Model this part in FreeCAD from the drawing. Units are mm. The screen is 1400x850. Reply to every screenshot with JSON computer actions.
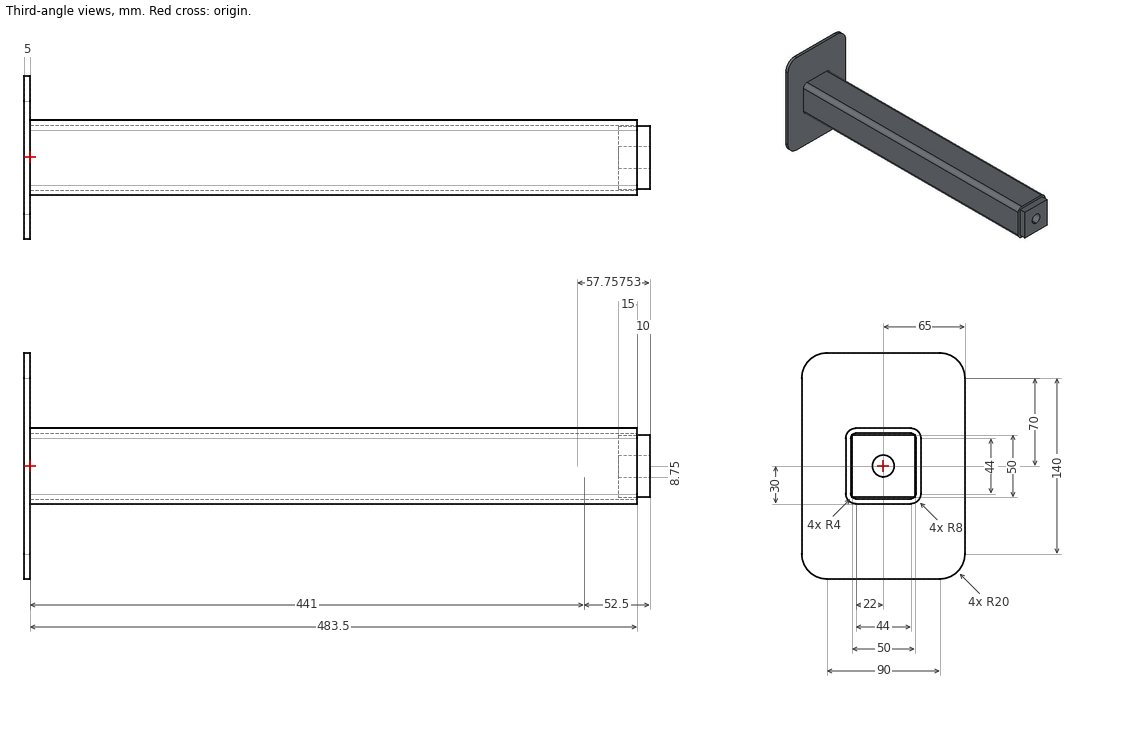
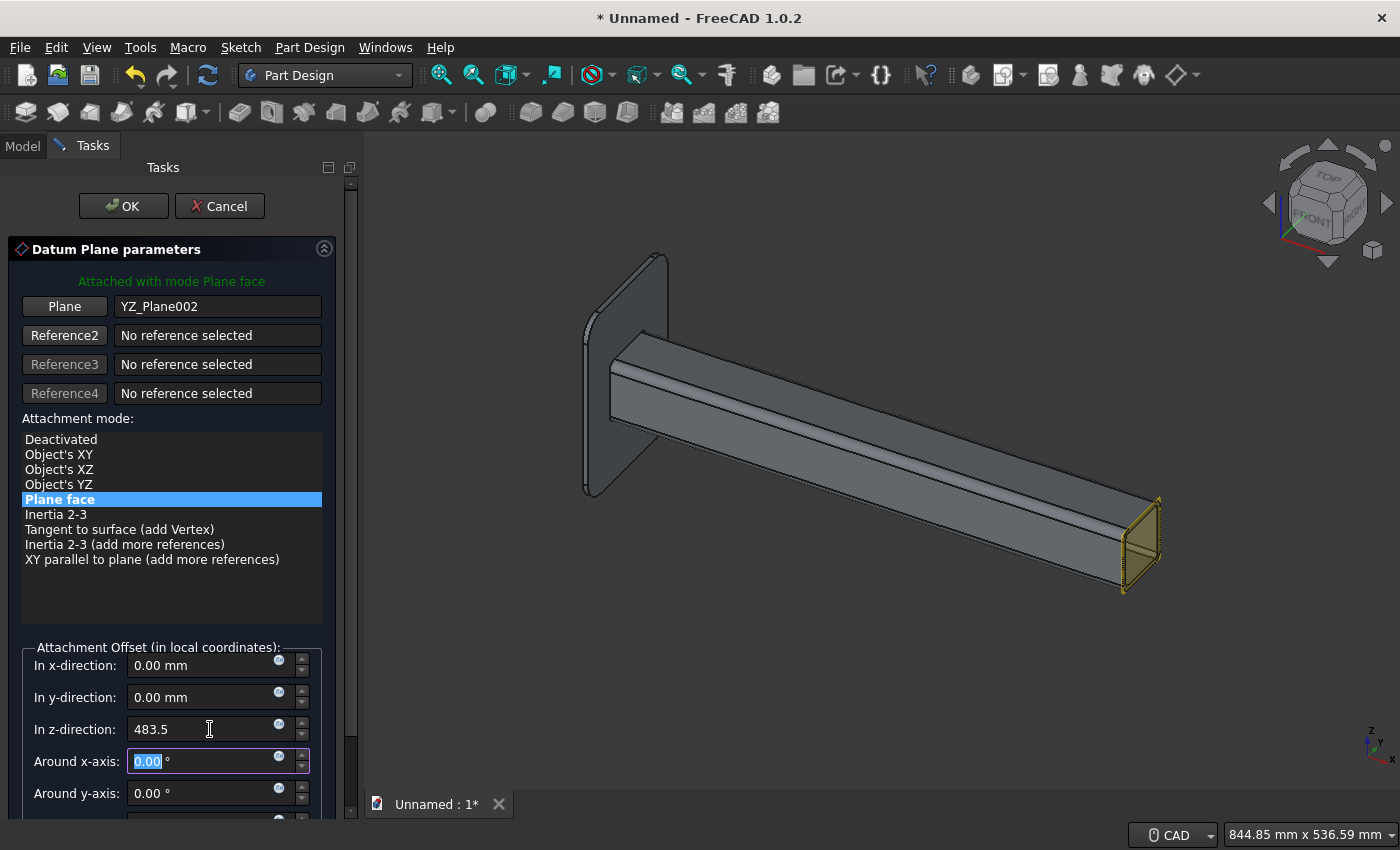
{"action": "left_click", "coordinate": [124, 206]}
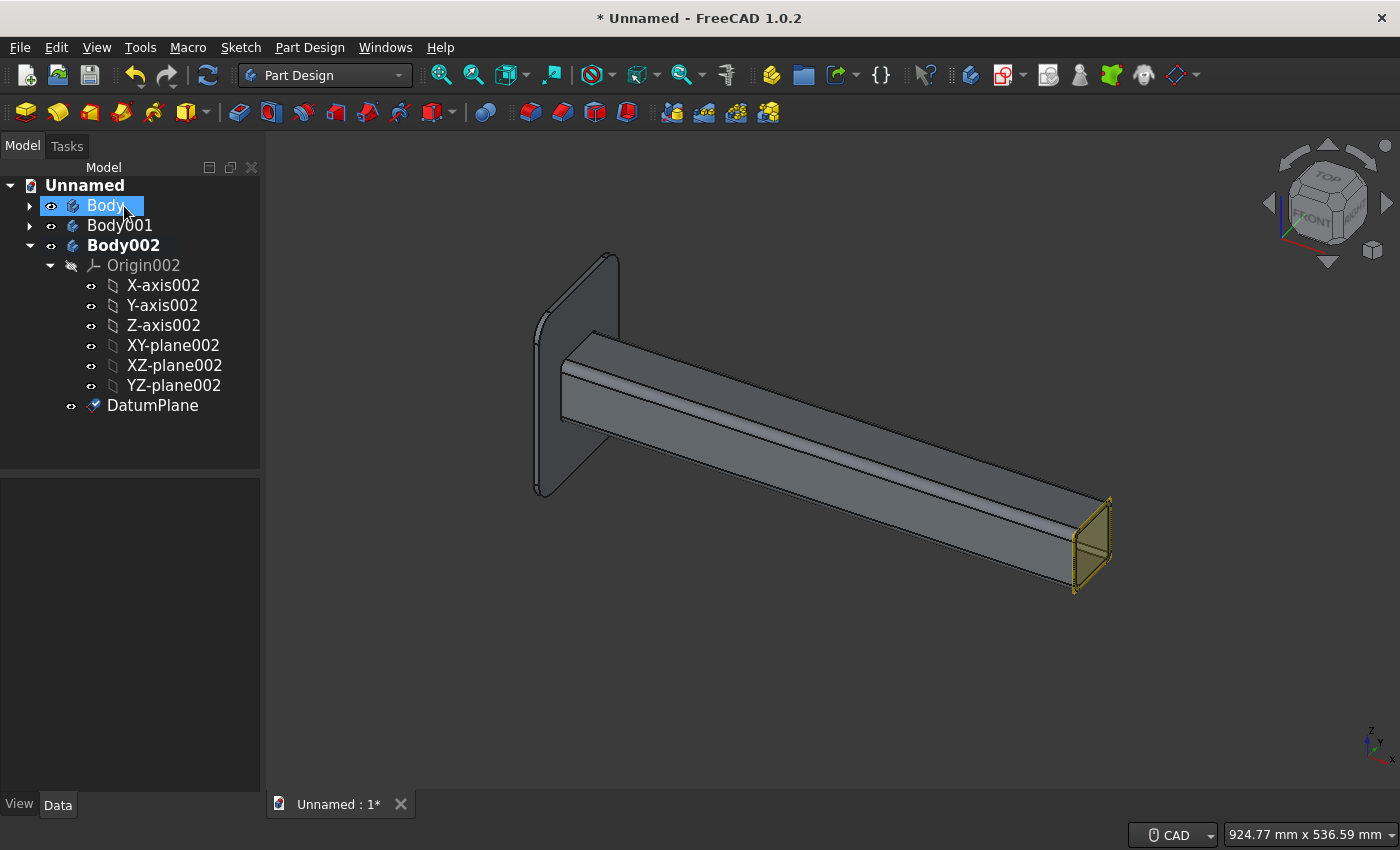
{"action": "left_click", "coordinate": [116, 406]}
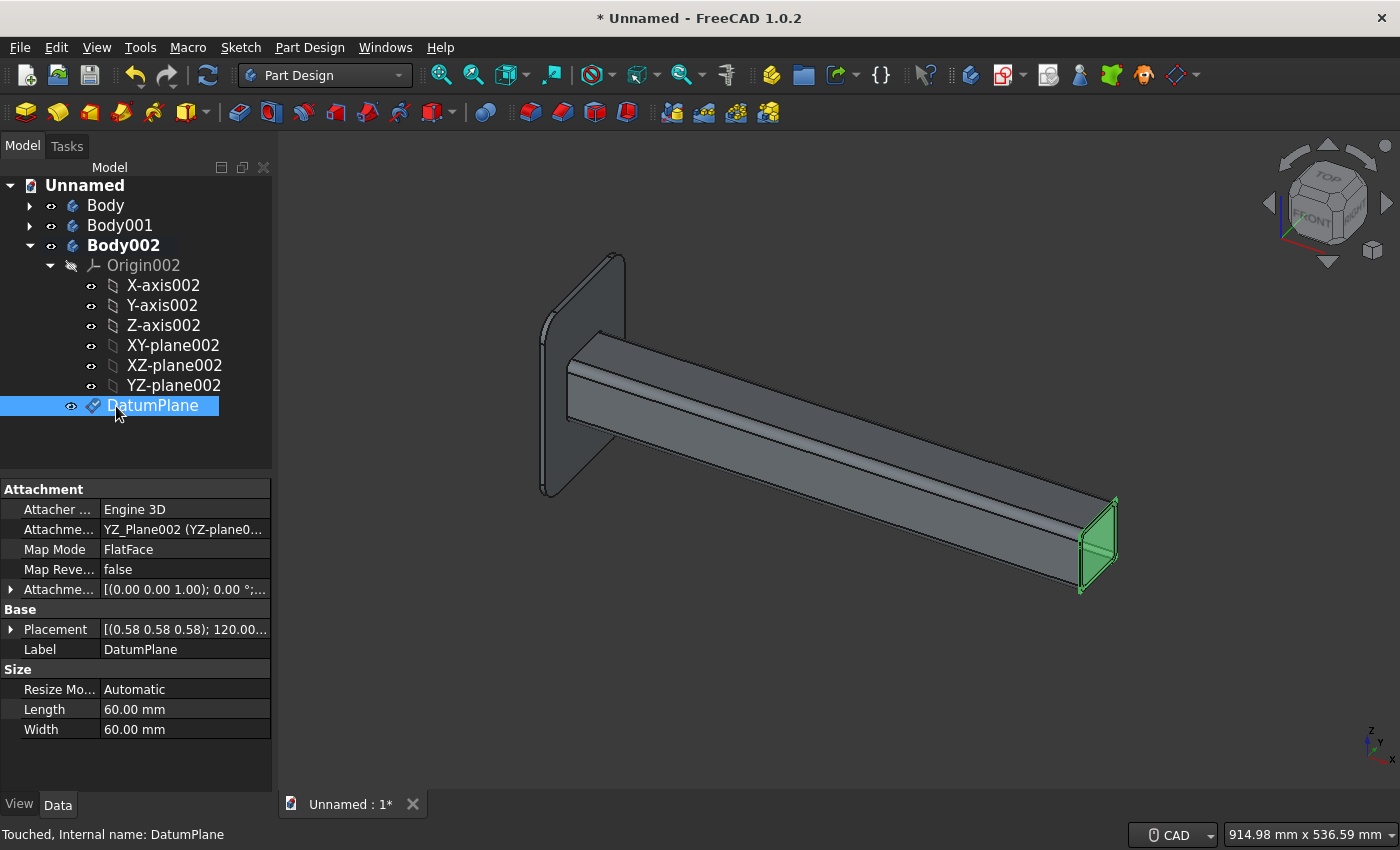
{"action": "left_click", "coordinate": [1004, 76]}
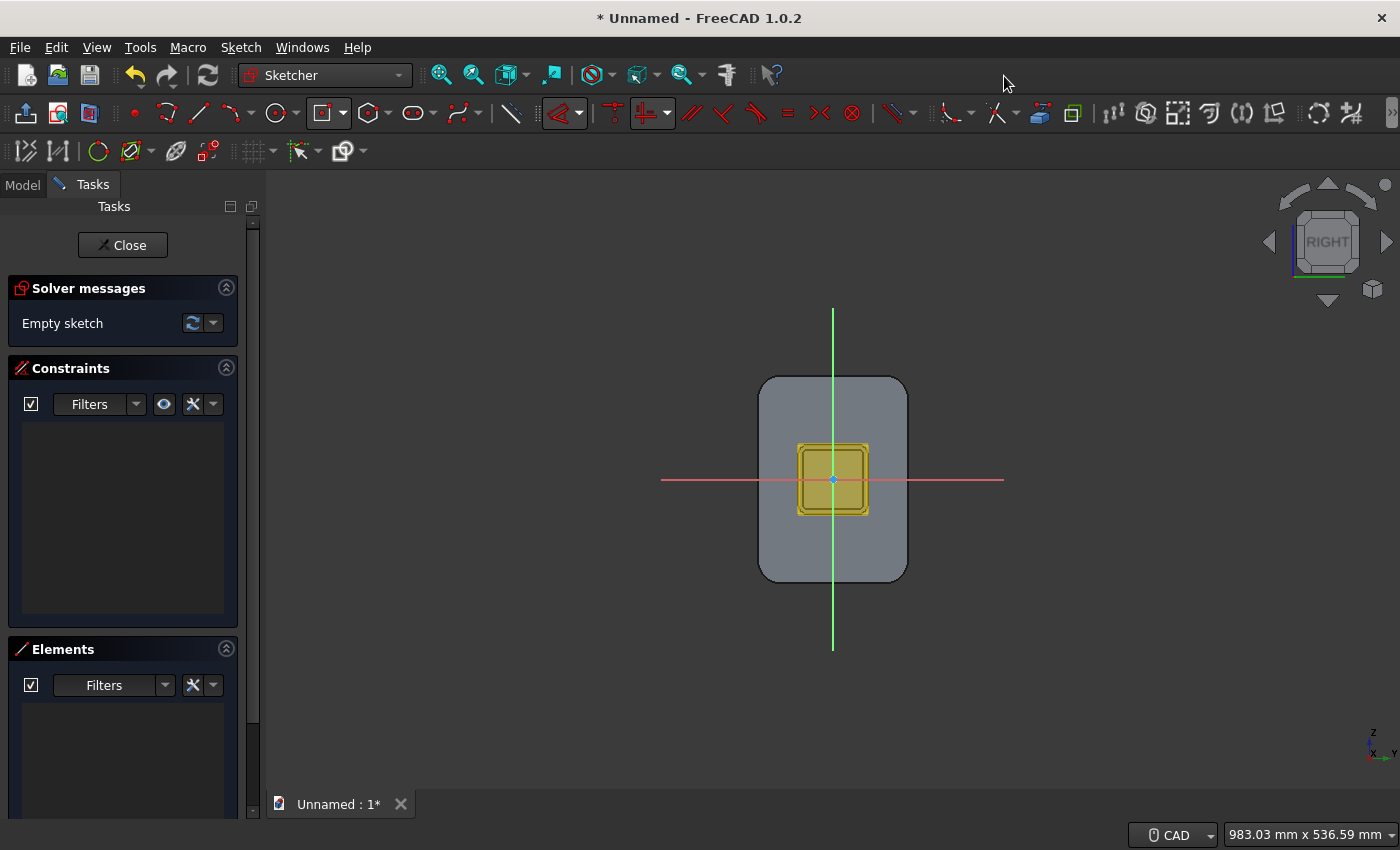
{"action": "scroll", "coordinate": [844, 480], "scroll_direction": "up", "scroll_amount": 10}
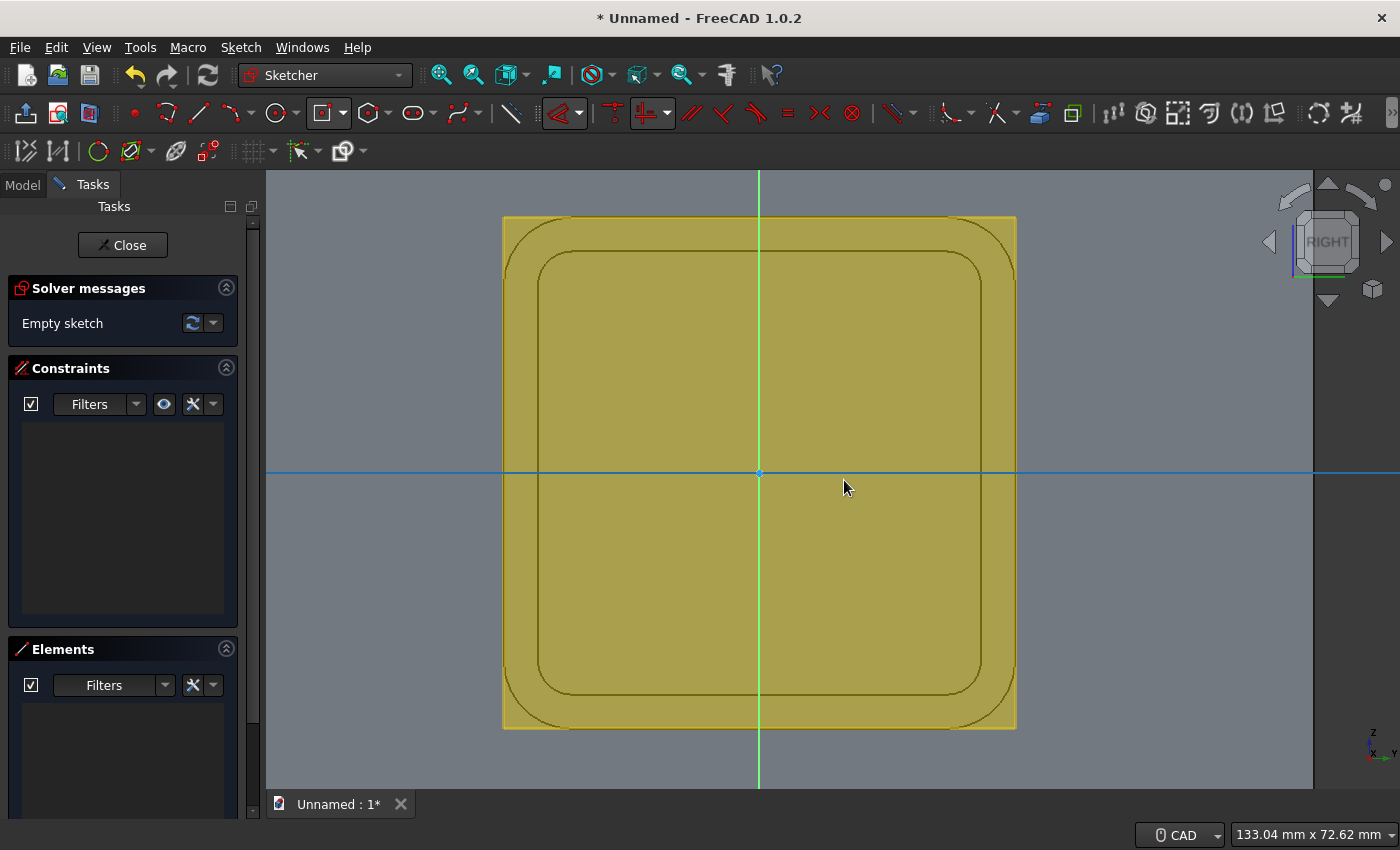
{"action": "key", "text": "g v"}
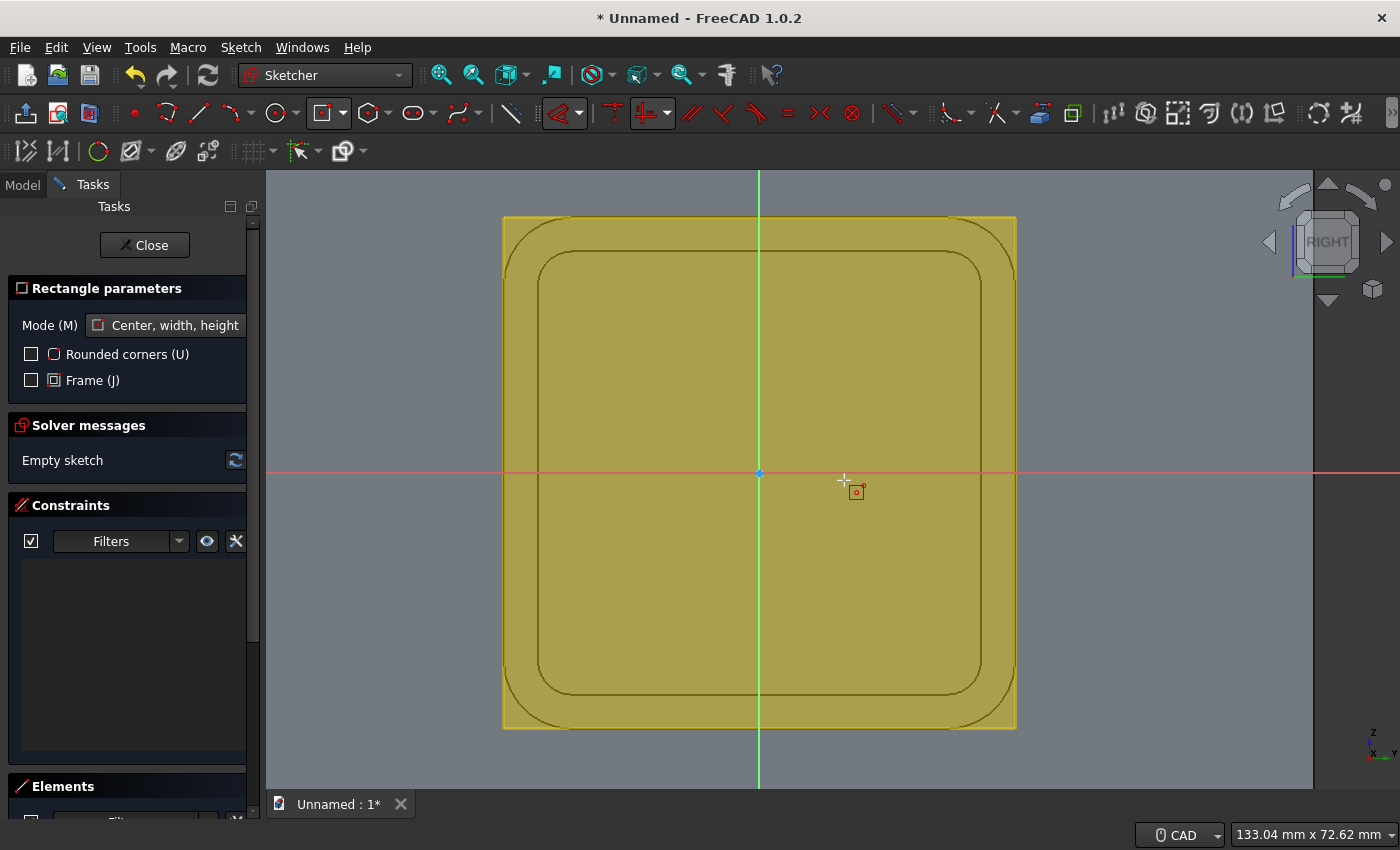
{"action": "left_click", "coordinate": [759, 473]}
{"action": "left_click", "coordinate": [973, 260]}
{"action": "key", "text": "Escape"}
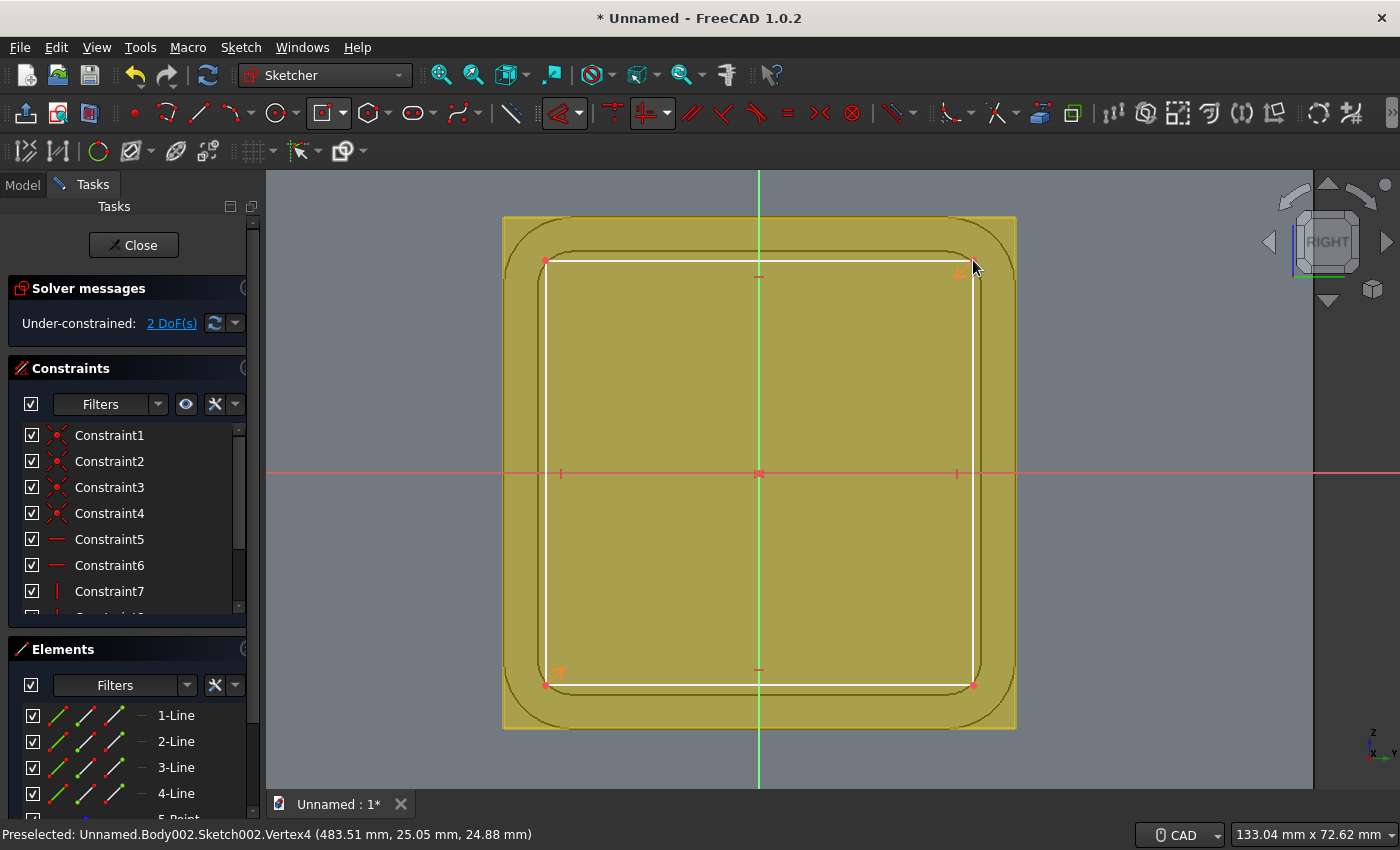
{"action": "left_click", "coordinate": [674, 685]}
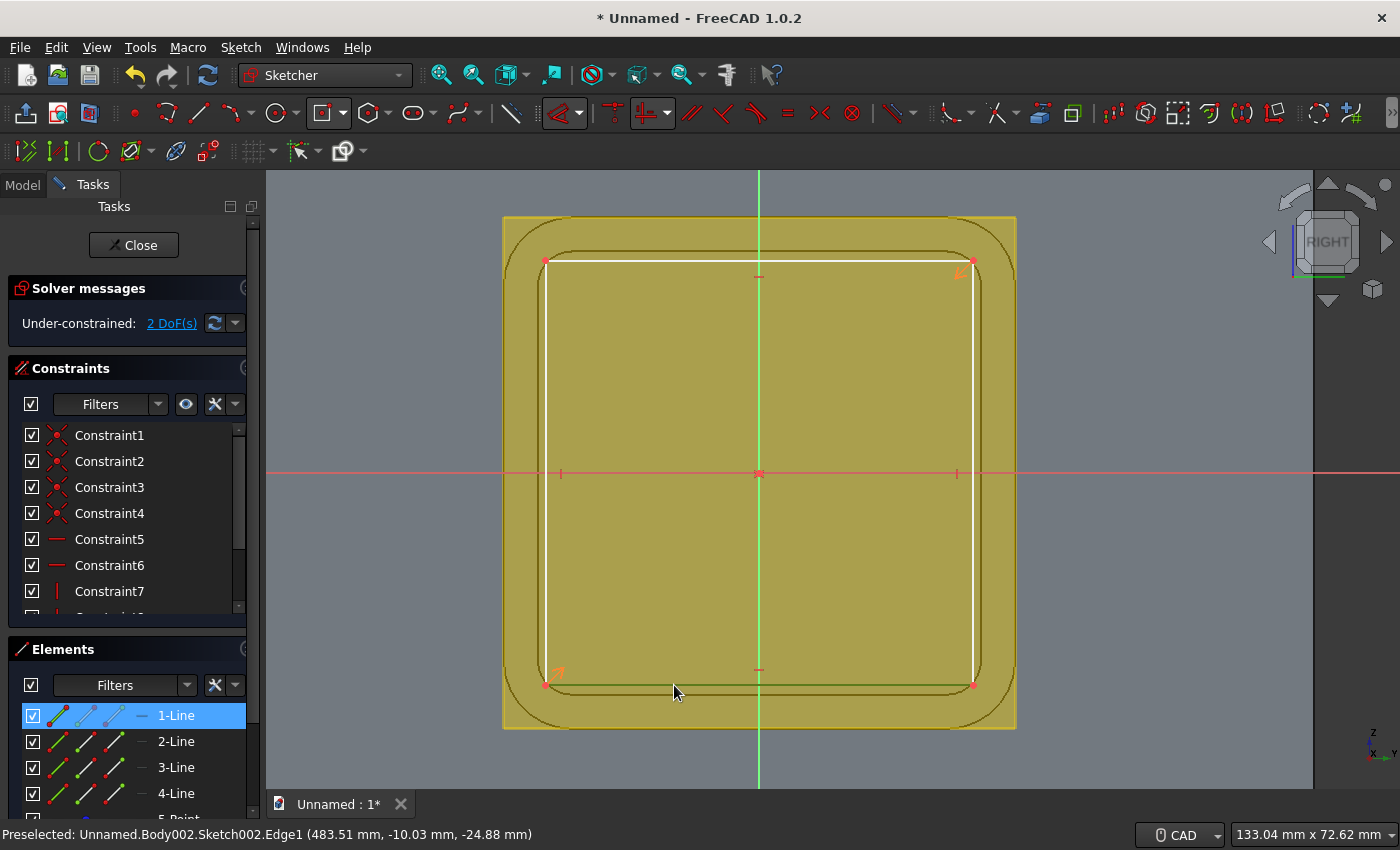
{"action": "left_click", "coordinate": [582, 114]}